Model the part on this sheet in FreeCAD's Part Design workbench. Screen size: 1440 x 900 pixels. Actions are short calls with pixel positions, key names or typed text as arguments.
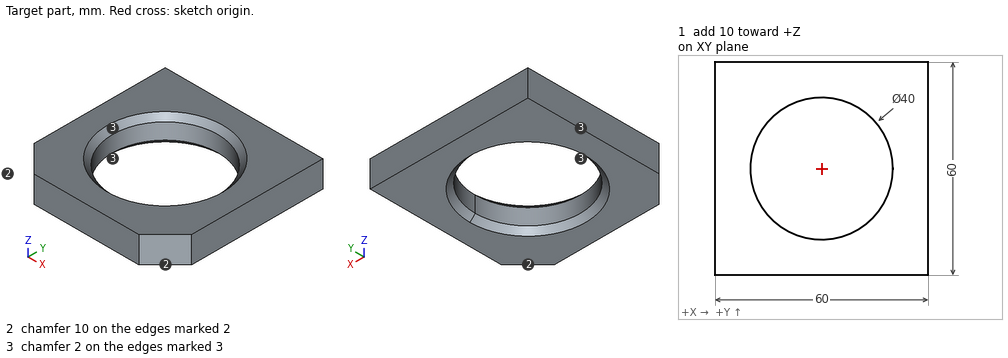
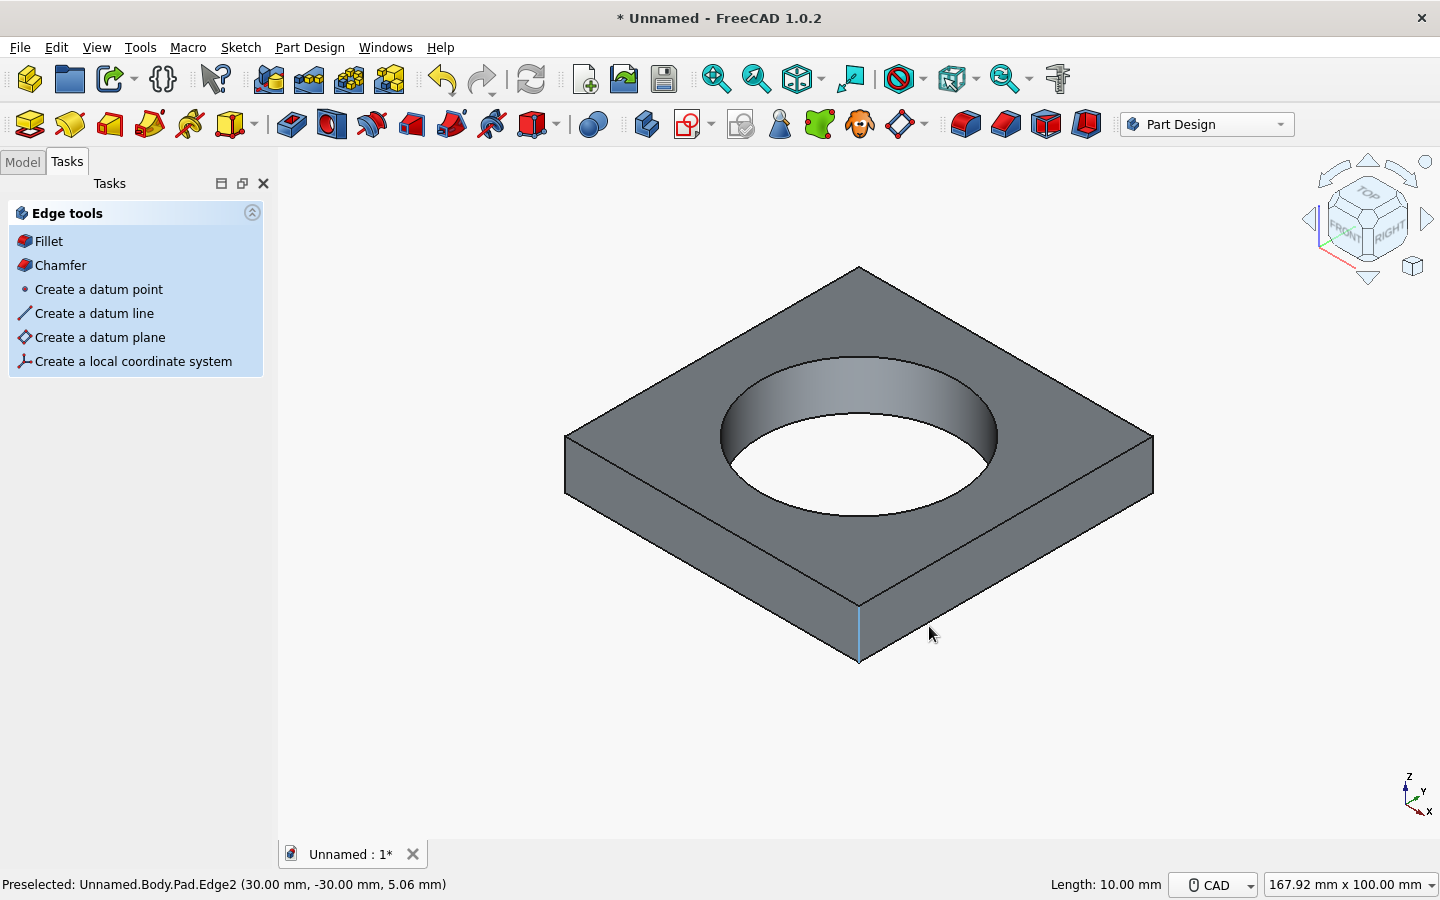
key(2)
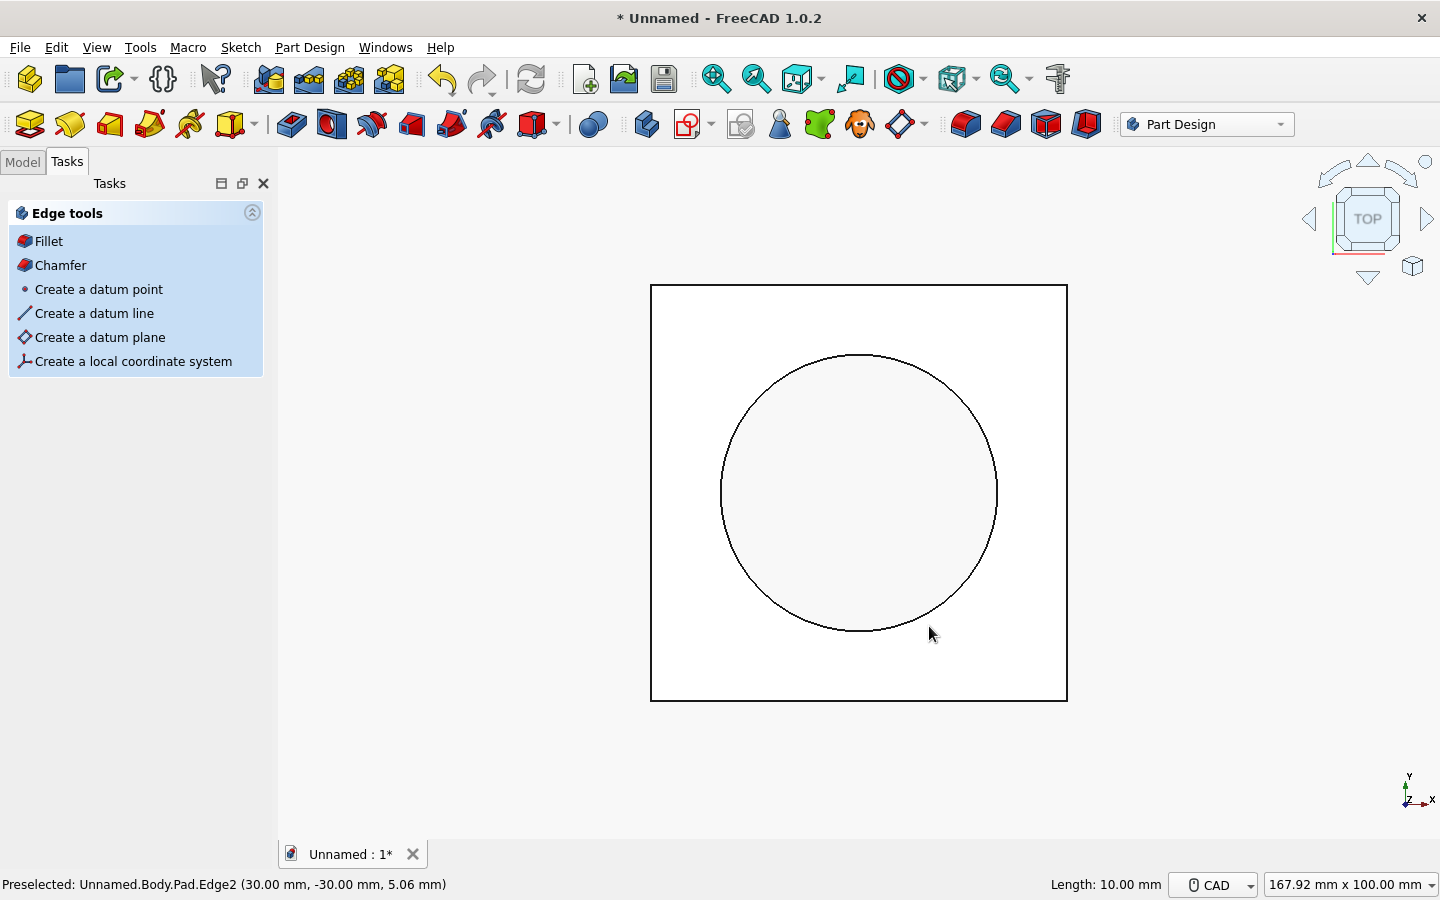
key(1)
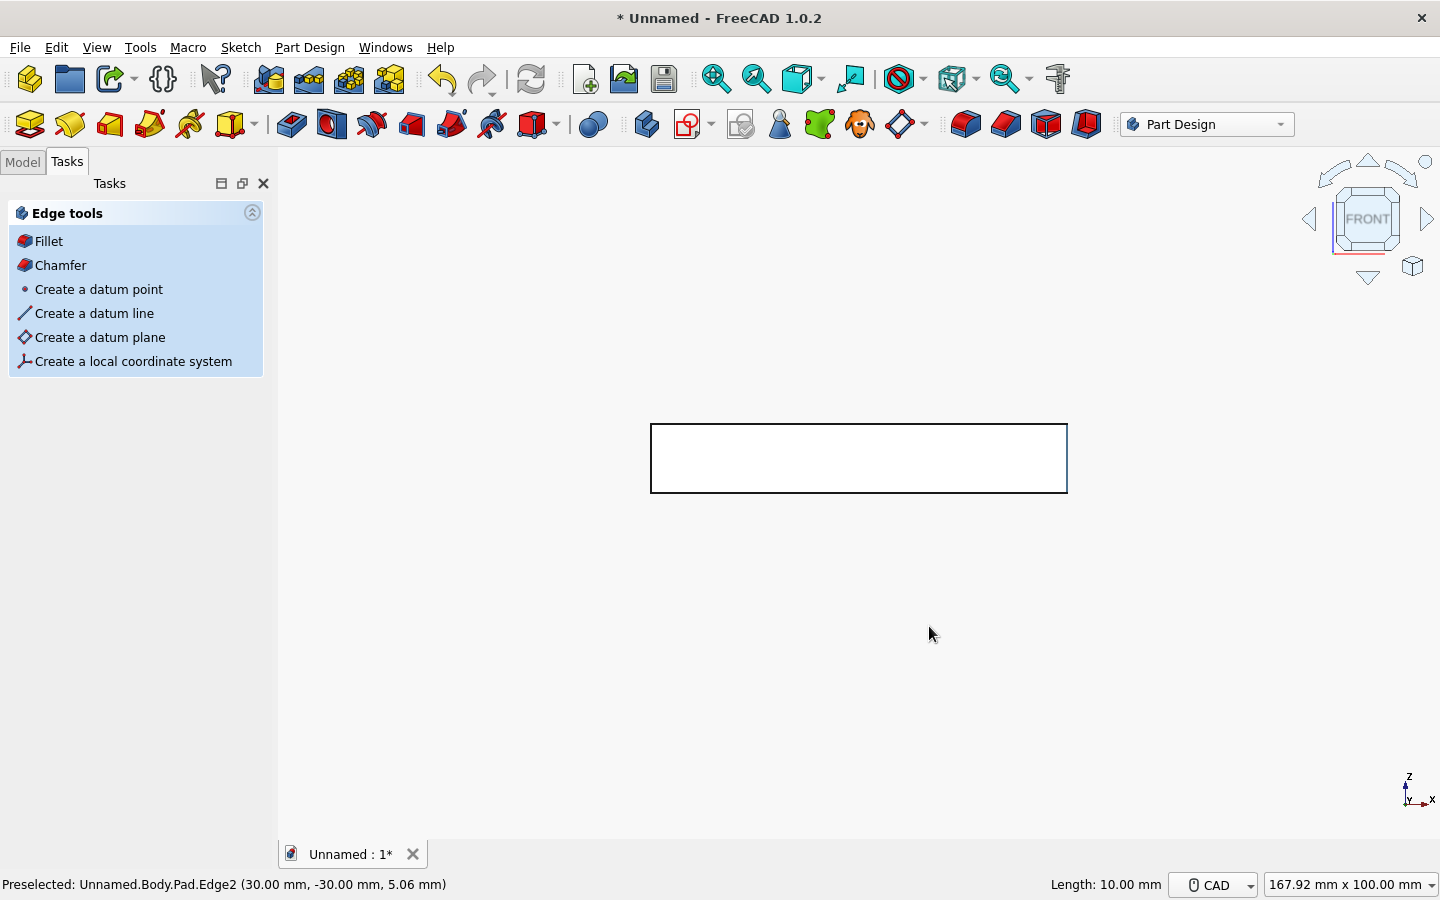
click(718, 80)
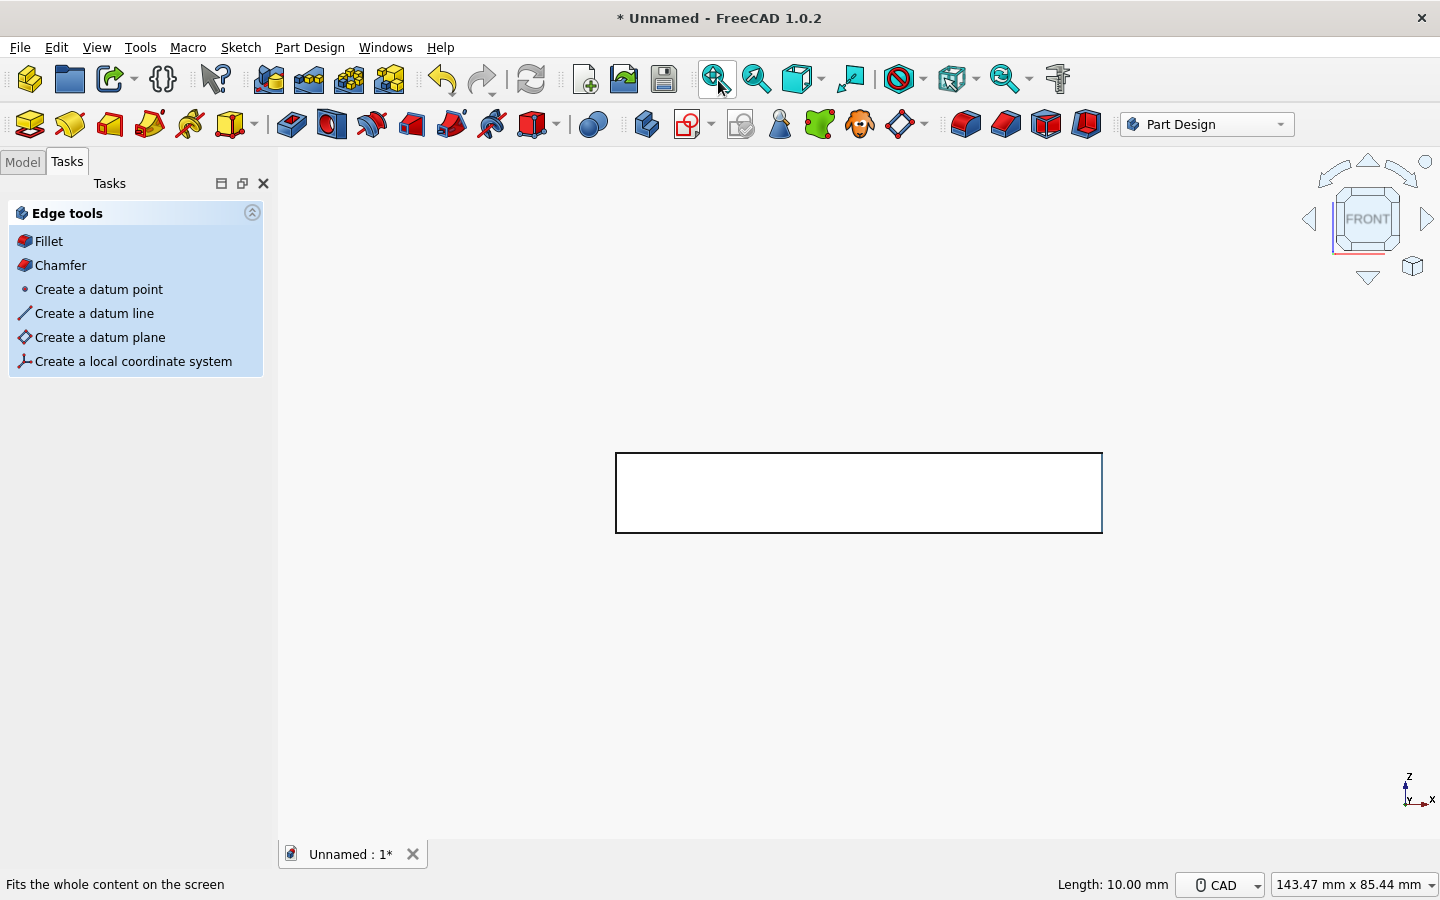
click(616, 492, ctrl)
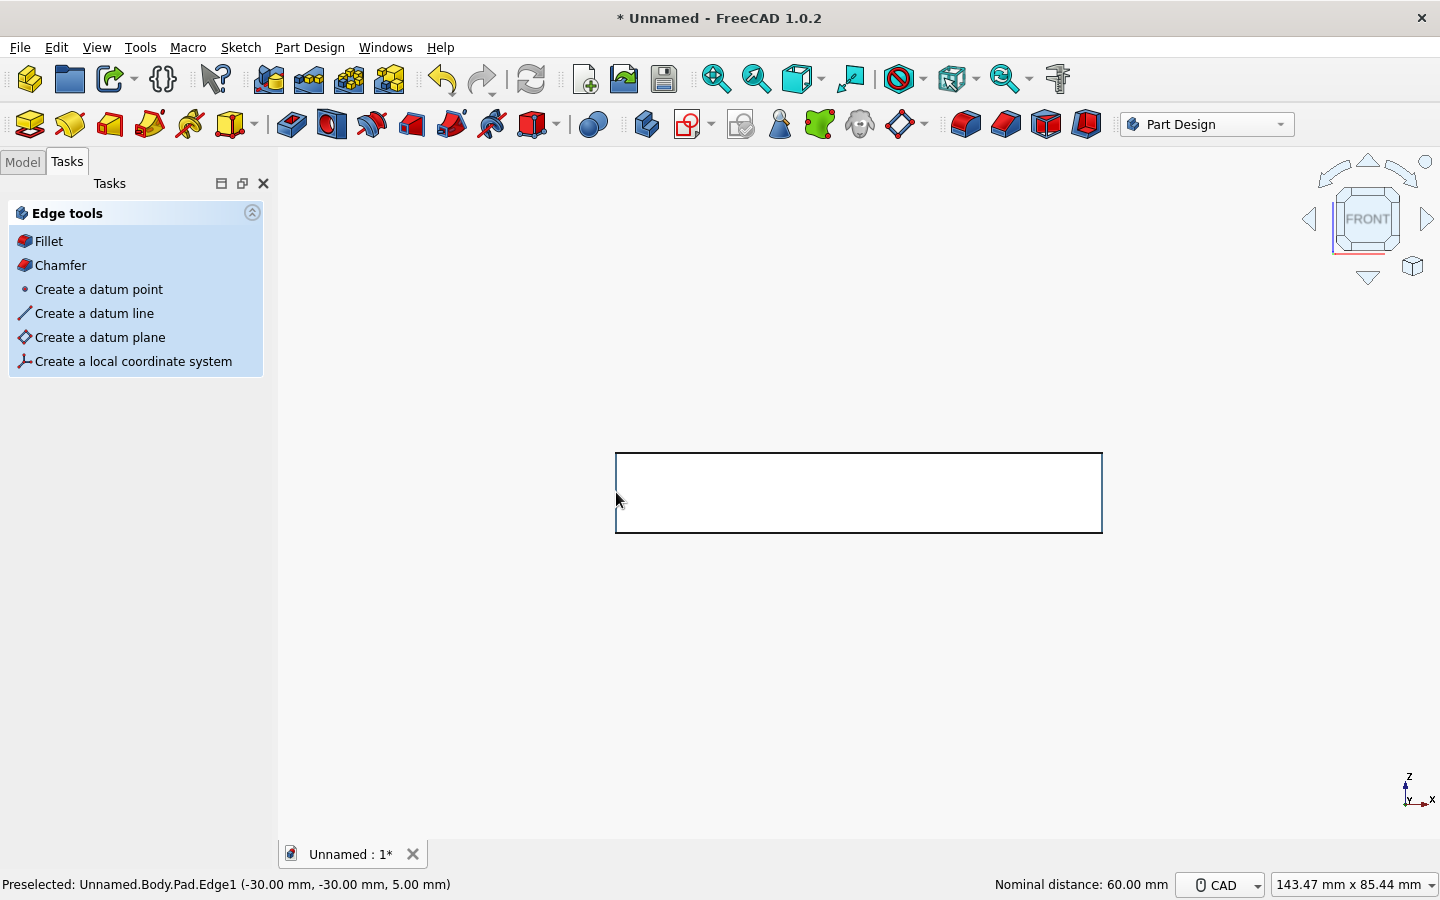
click(1006, 124)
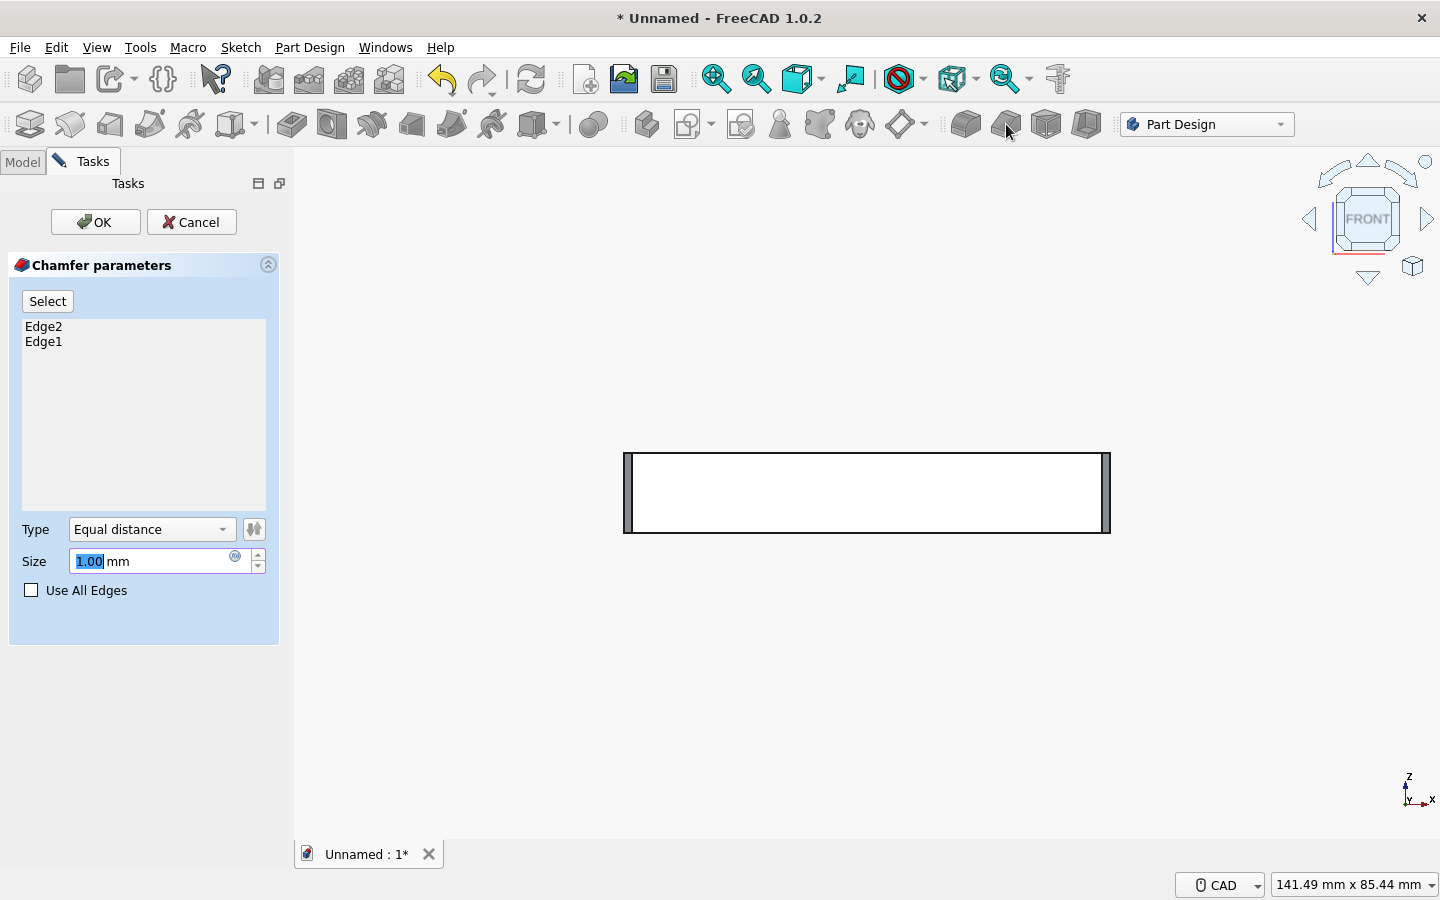
text(10)
key(Tab)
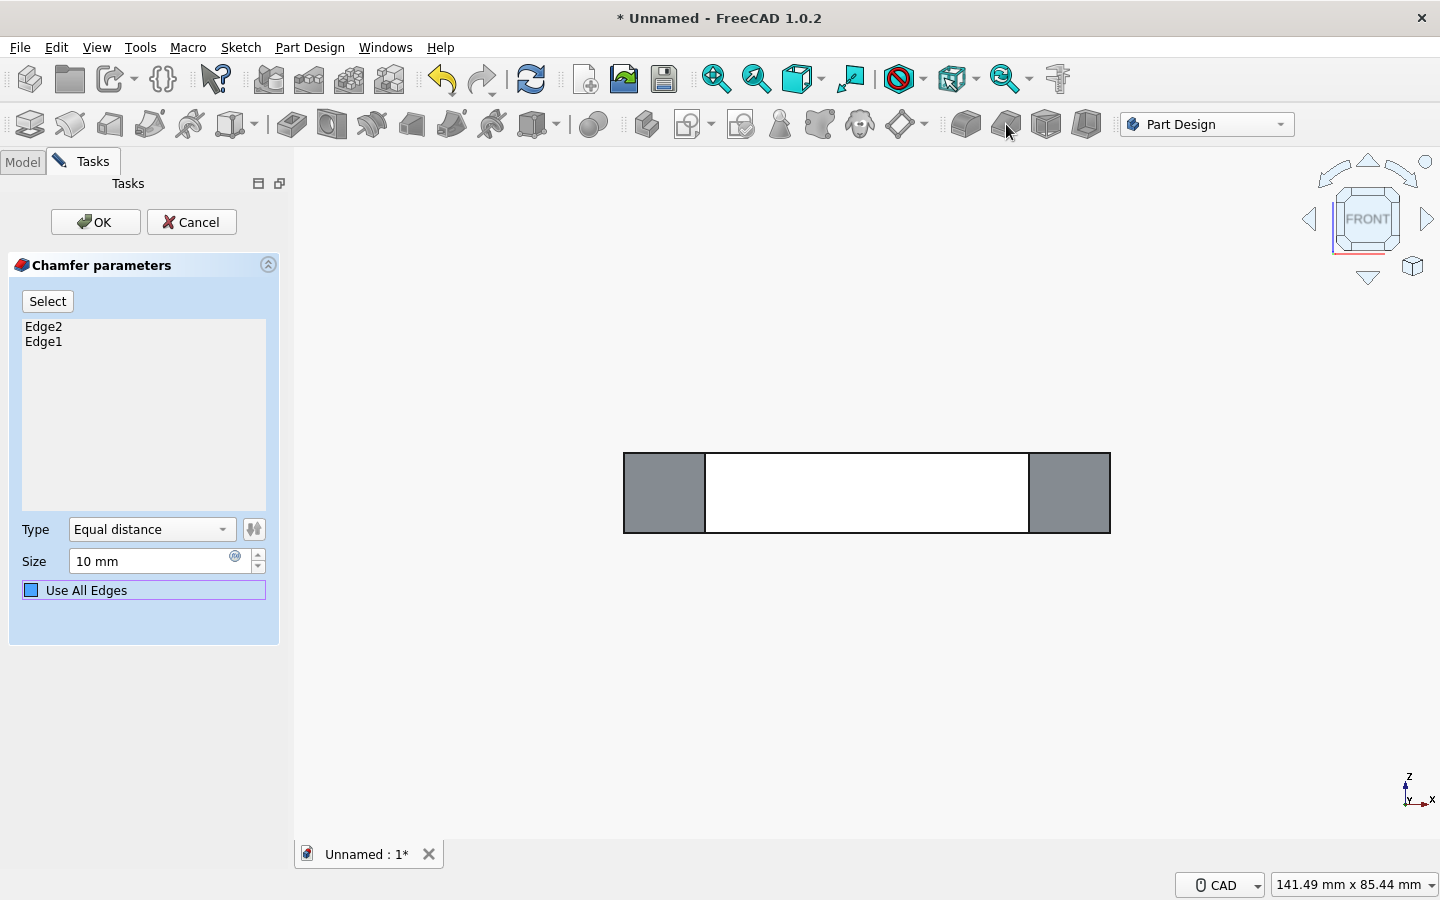
click(96, 222)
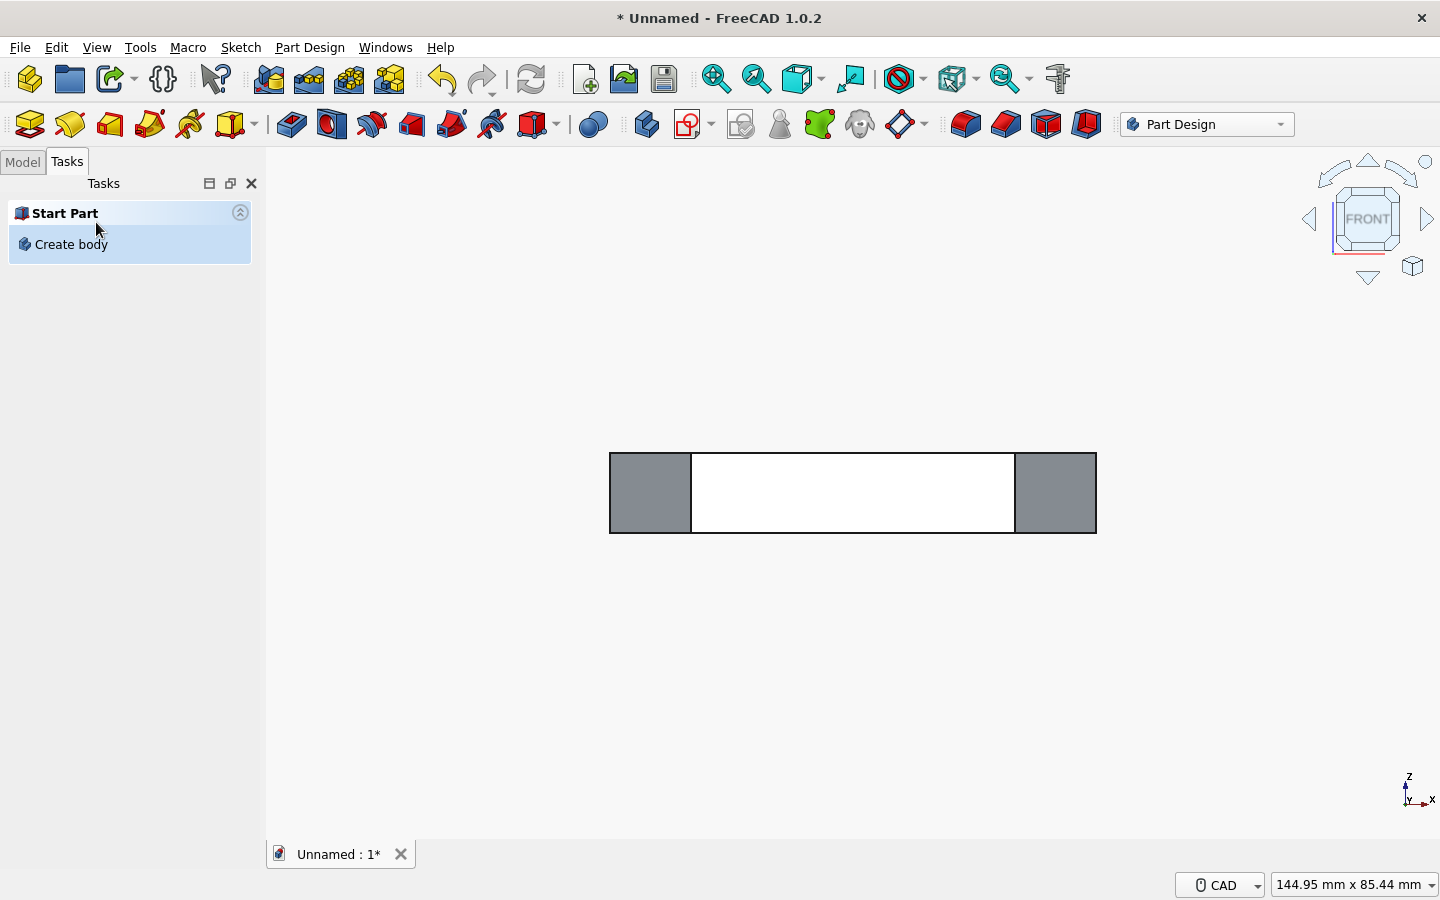
click(718, 80)